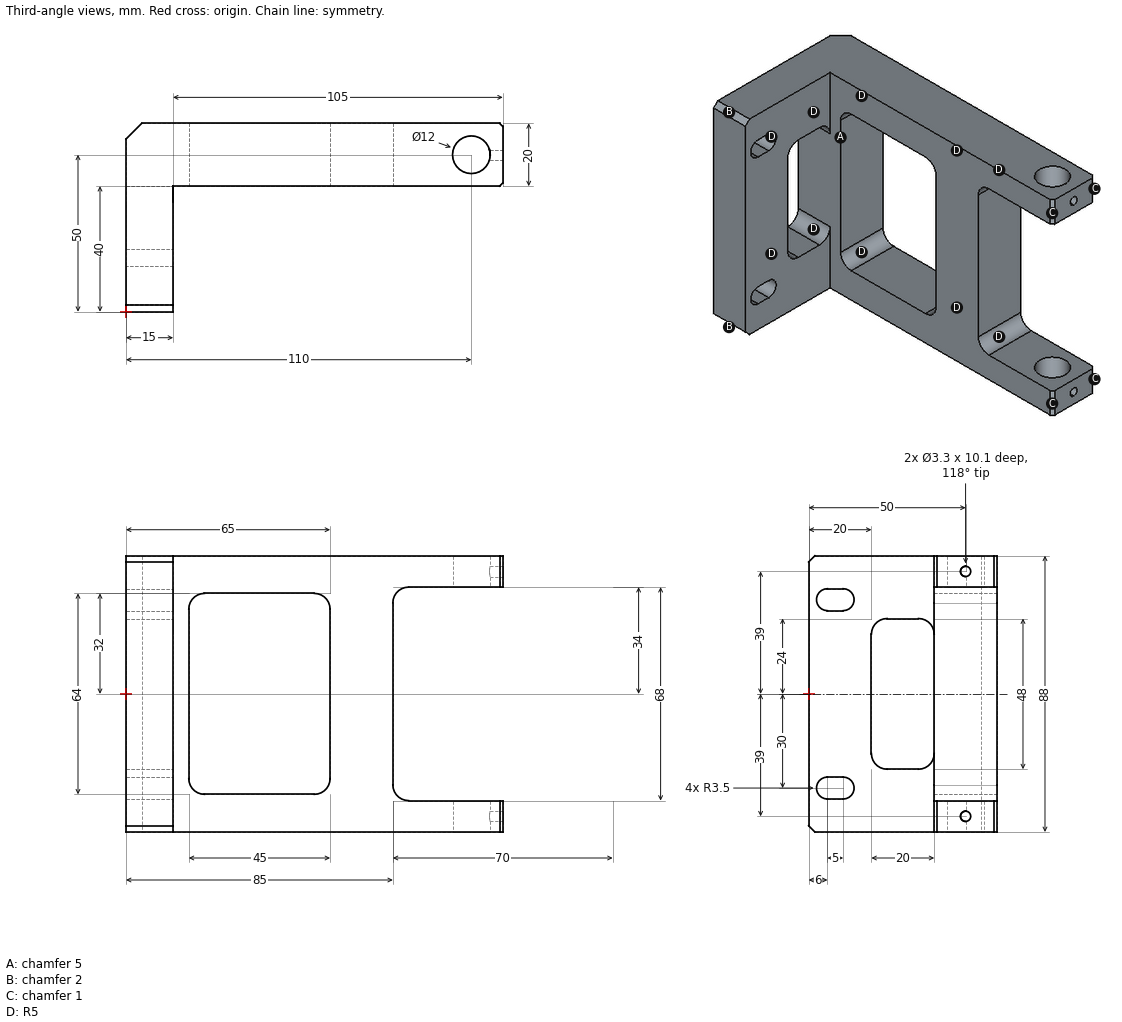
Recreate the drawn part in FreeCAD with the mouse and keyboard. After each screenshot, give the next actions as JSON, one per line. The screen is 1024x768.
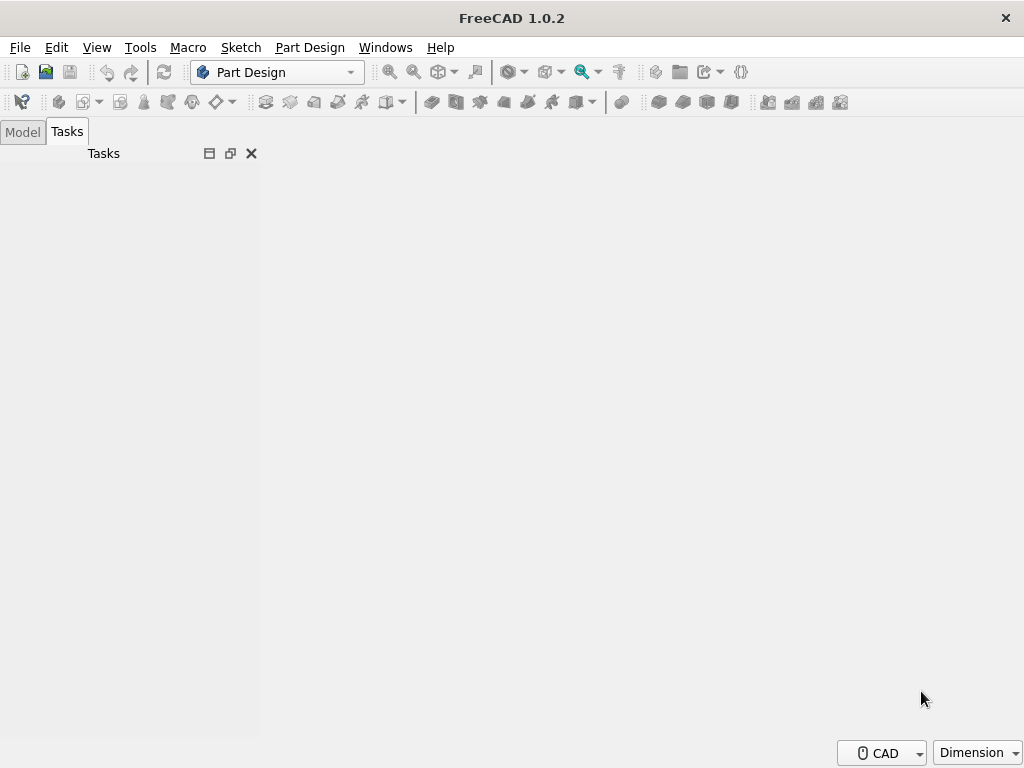
{"action": "left_click", "coordinate": [22, 72]}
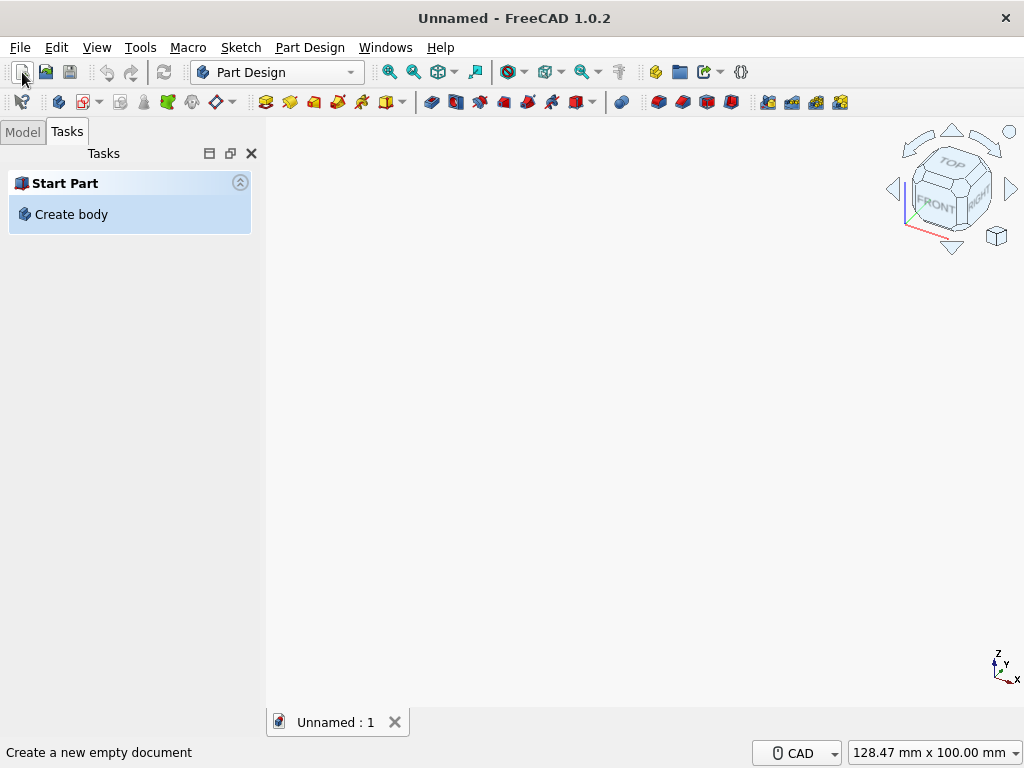
{"action": "left_click", "coordinate": [84, 102]}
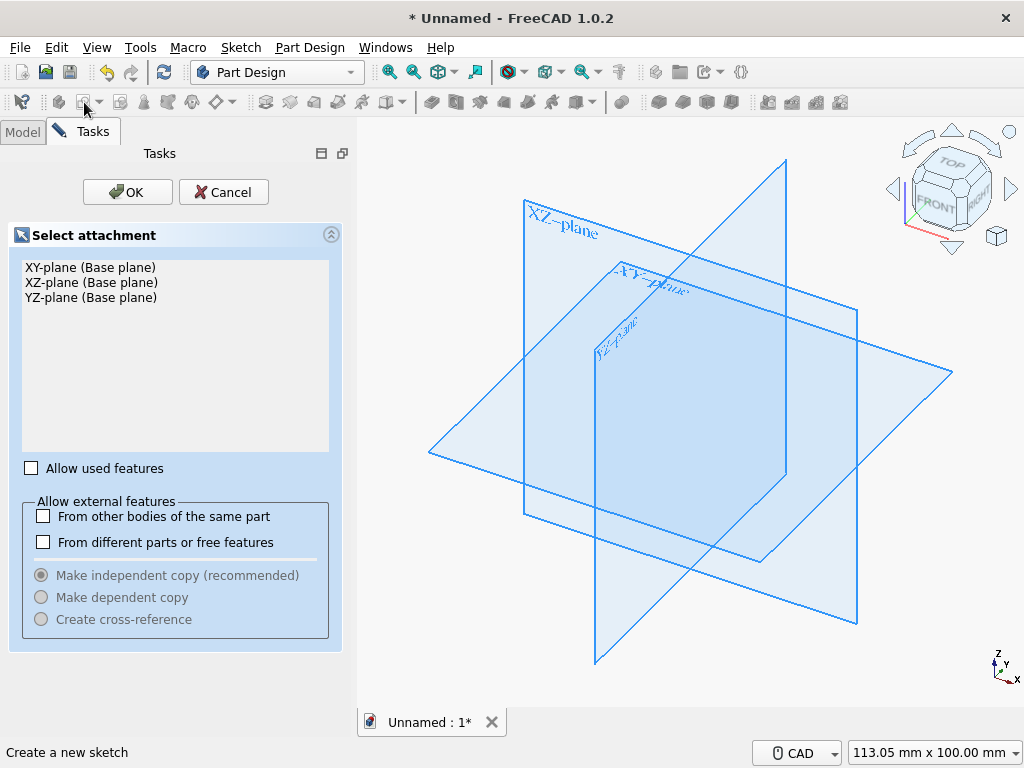
{"action": "left_click", "coordinate": [82, 268]}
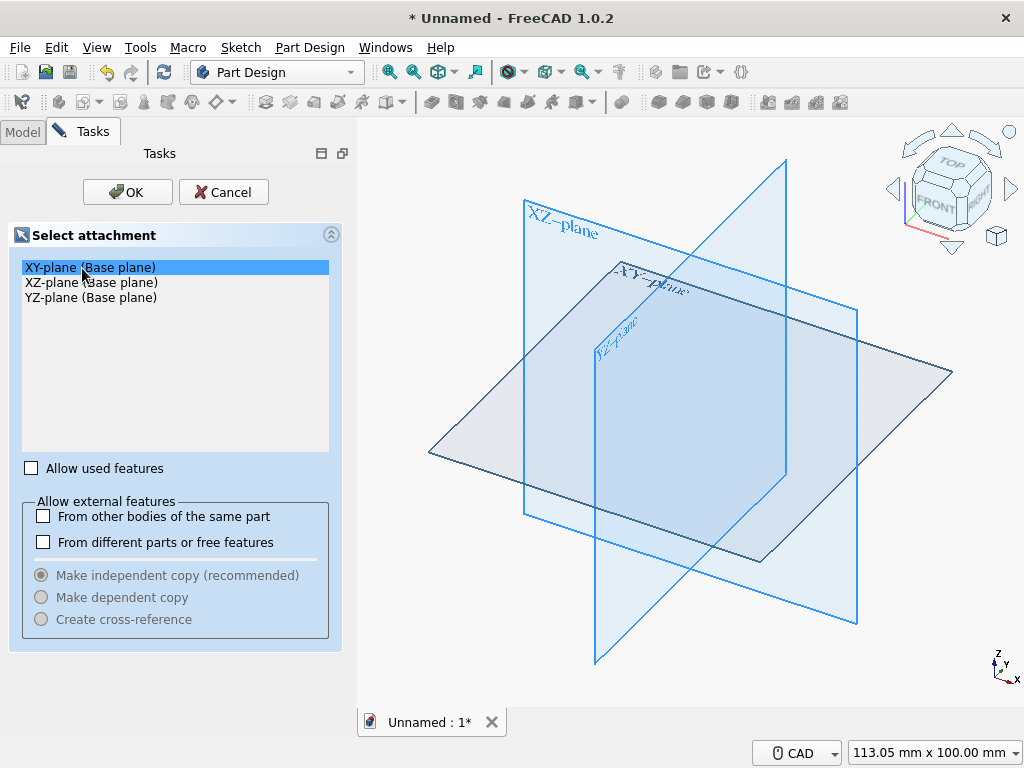
{"action": "left_click", "coordinate": [128, 192]}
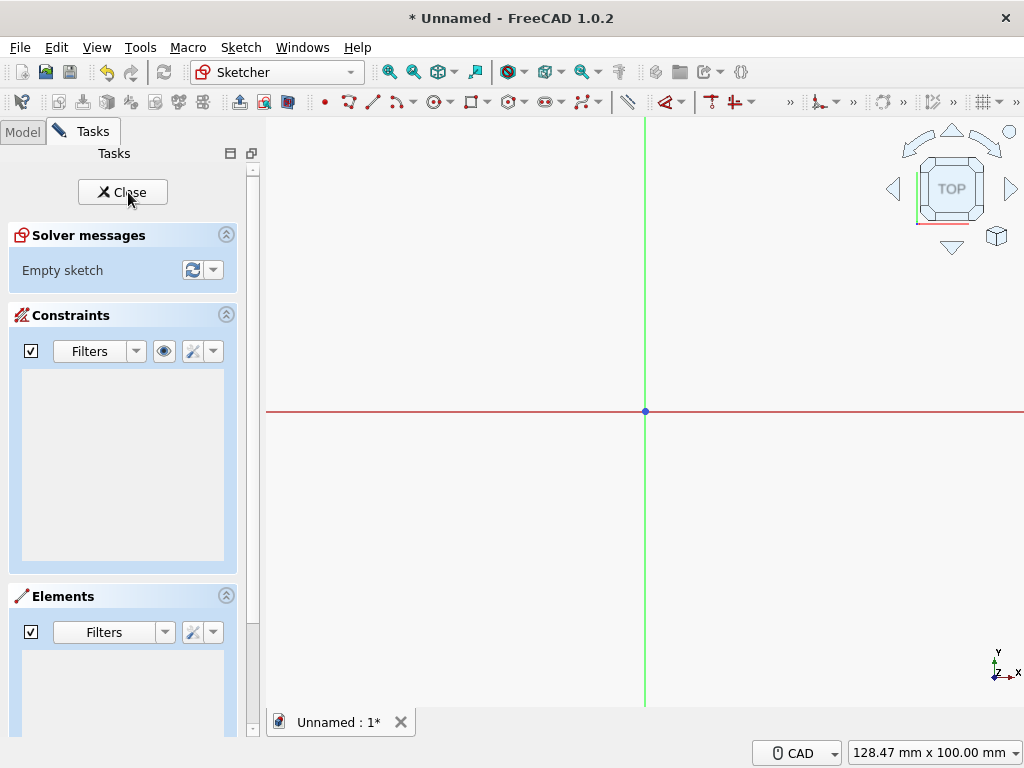
{"action": "scroll", "coordinate": [294, 556], "scroll_direction": "down", "scroll_amount": 4}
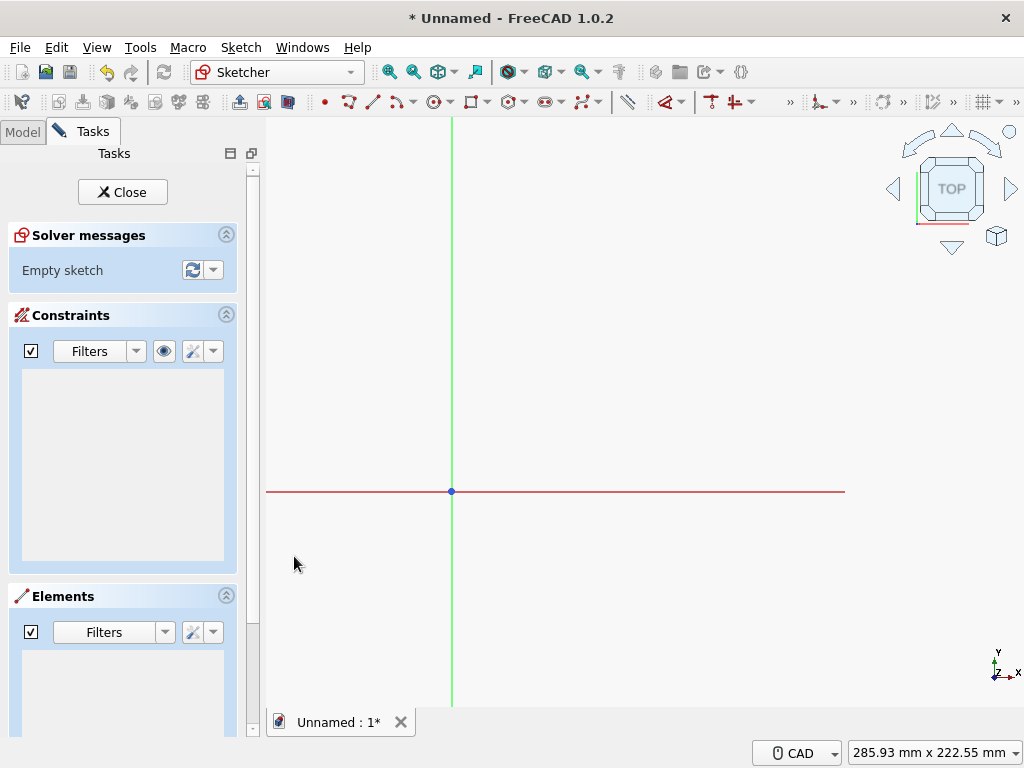
{"action": "key", "text": "g m"}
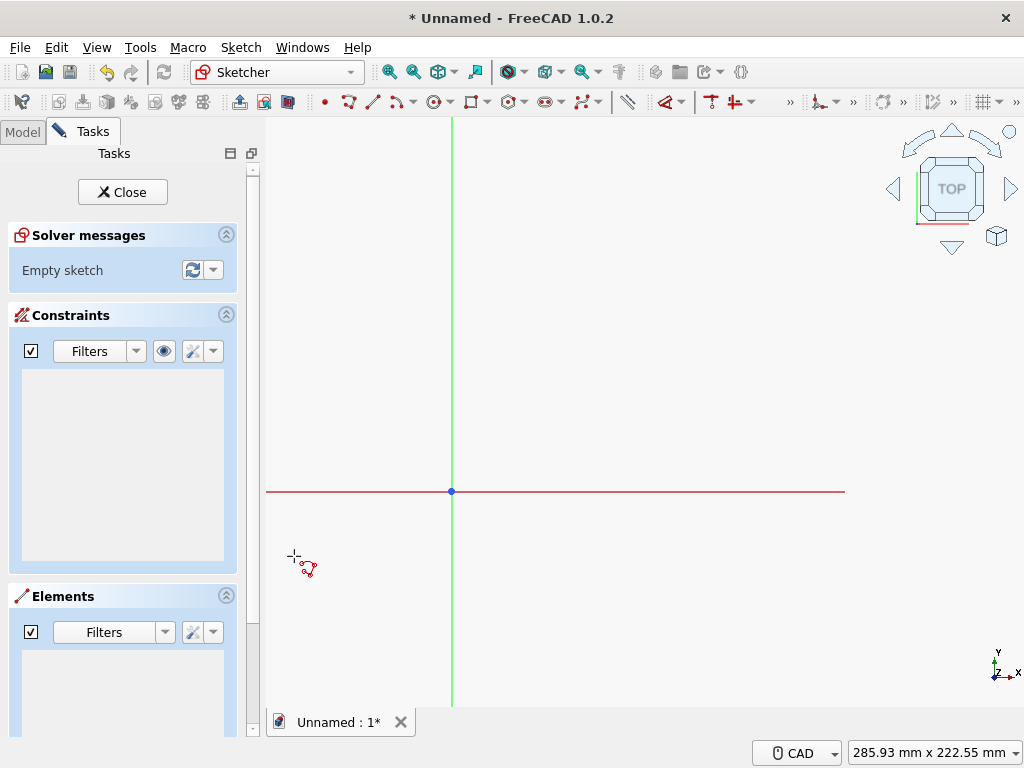
{"action": "left_click", "coordinate": [452, 492]}
{"action": "left_click", "coordinate": [492, 483]}
{"action": "left_click", "coordinate": [492, 386]}
{"action": "left_click", "coordinate": [770, 386]}
{"action": "left_click", "coordinate": [770, 333]}
{"action": "left_click", "coordinate": [461, 333]}
{"action": "left_click", "coordinate": [452, 492]}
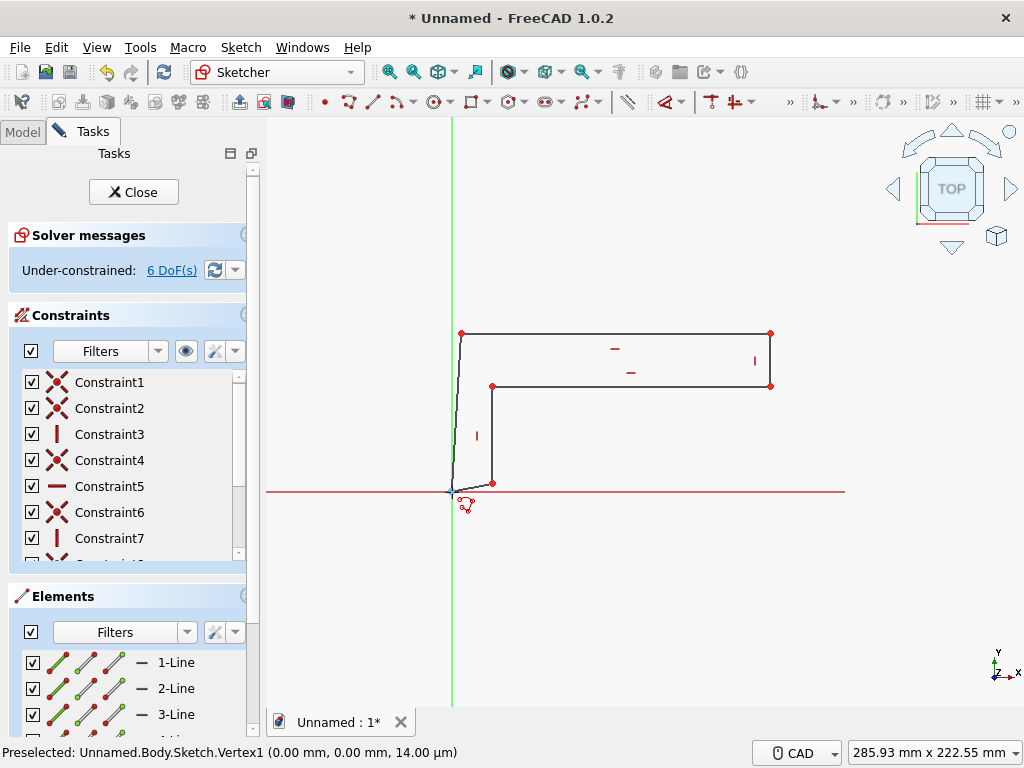
{"action": "left_click", "coordinate": [434, 102]}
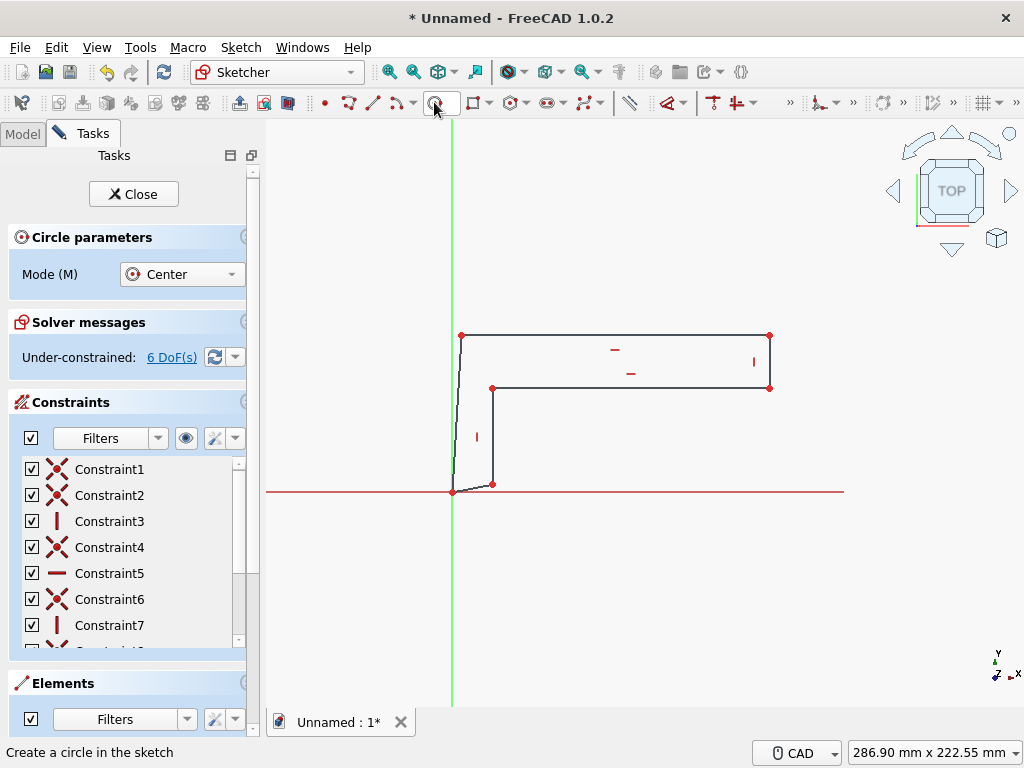
{"action": "scroll", "coordinate": [743, 360], "scroll_direction": "up", "scroll_amount": 2}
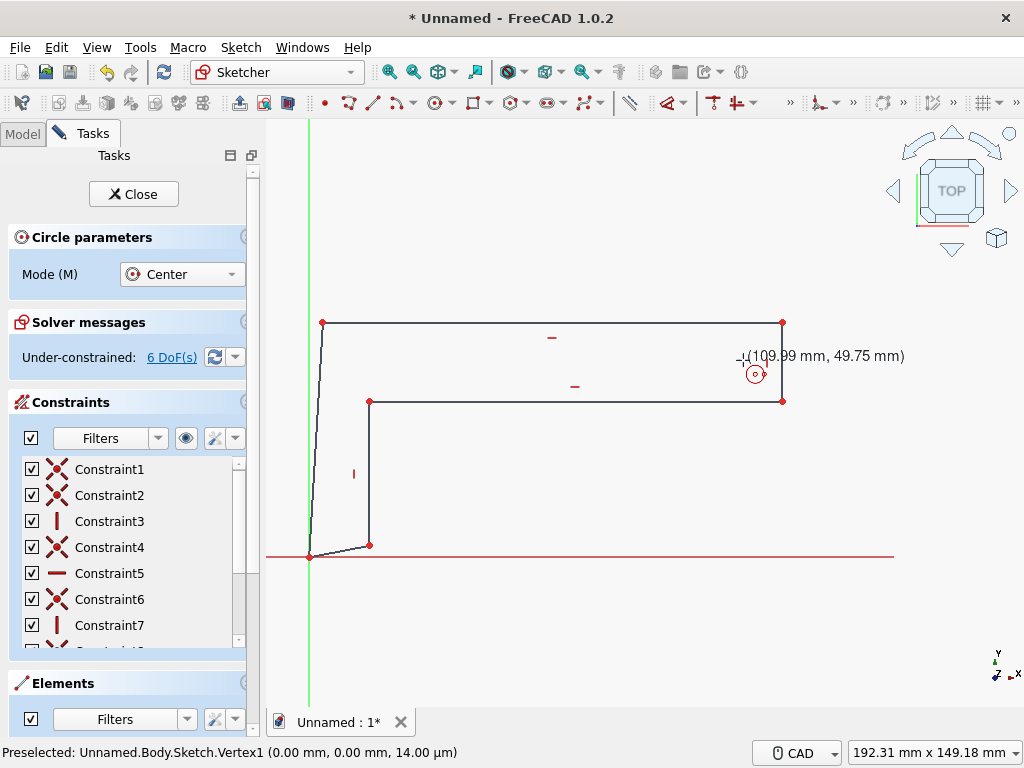
{"action": "left_click", "coordinate": [743, 360]}
{"action": "mouse_move", "coordinate": [759, 344]}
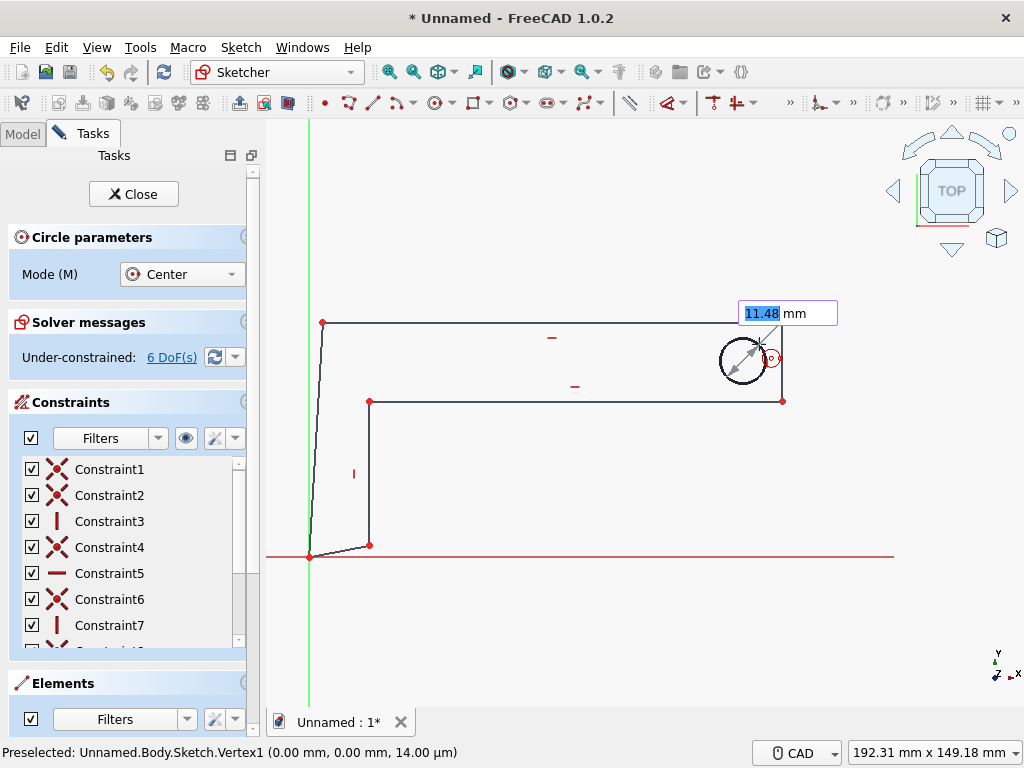
{"action": "type", "text": "12"}
{"action": "key", "text": "Return"}
{"action": "key", "text": "Escape"}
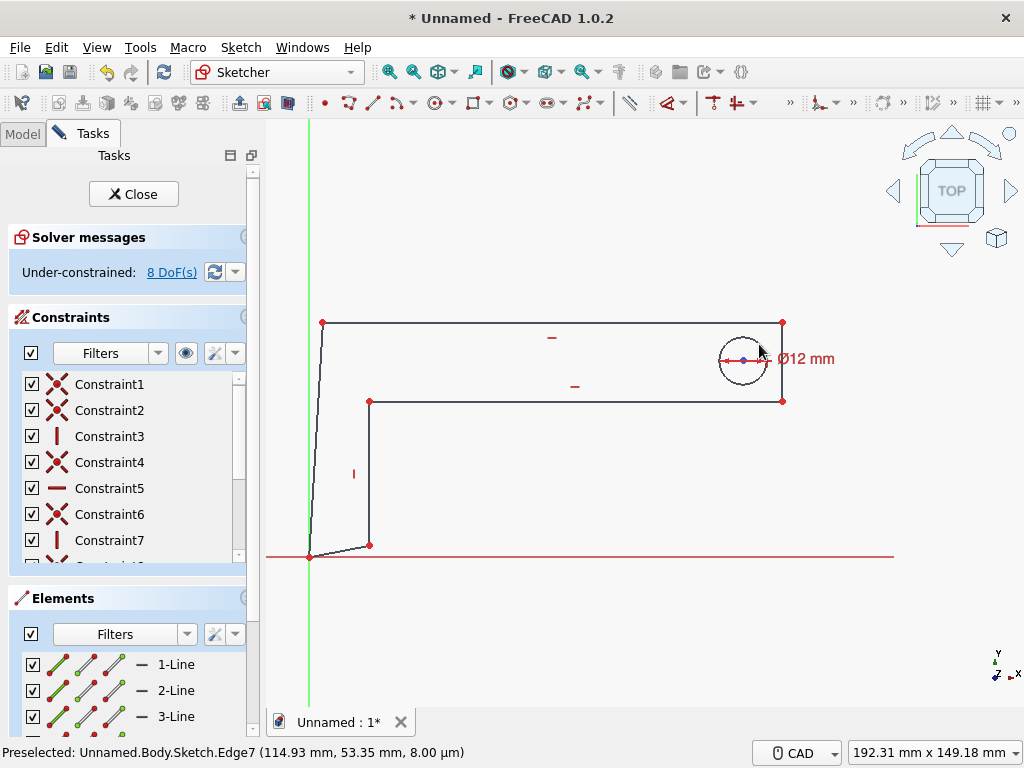
{"action": "left_click", "coordinate": [327, 554]}